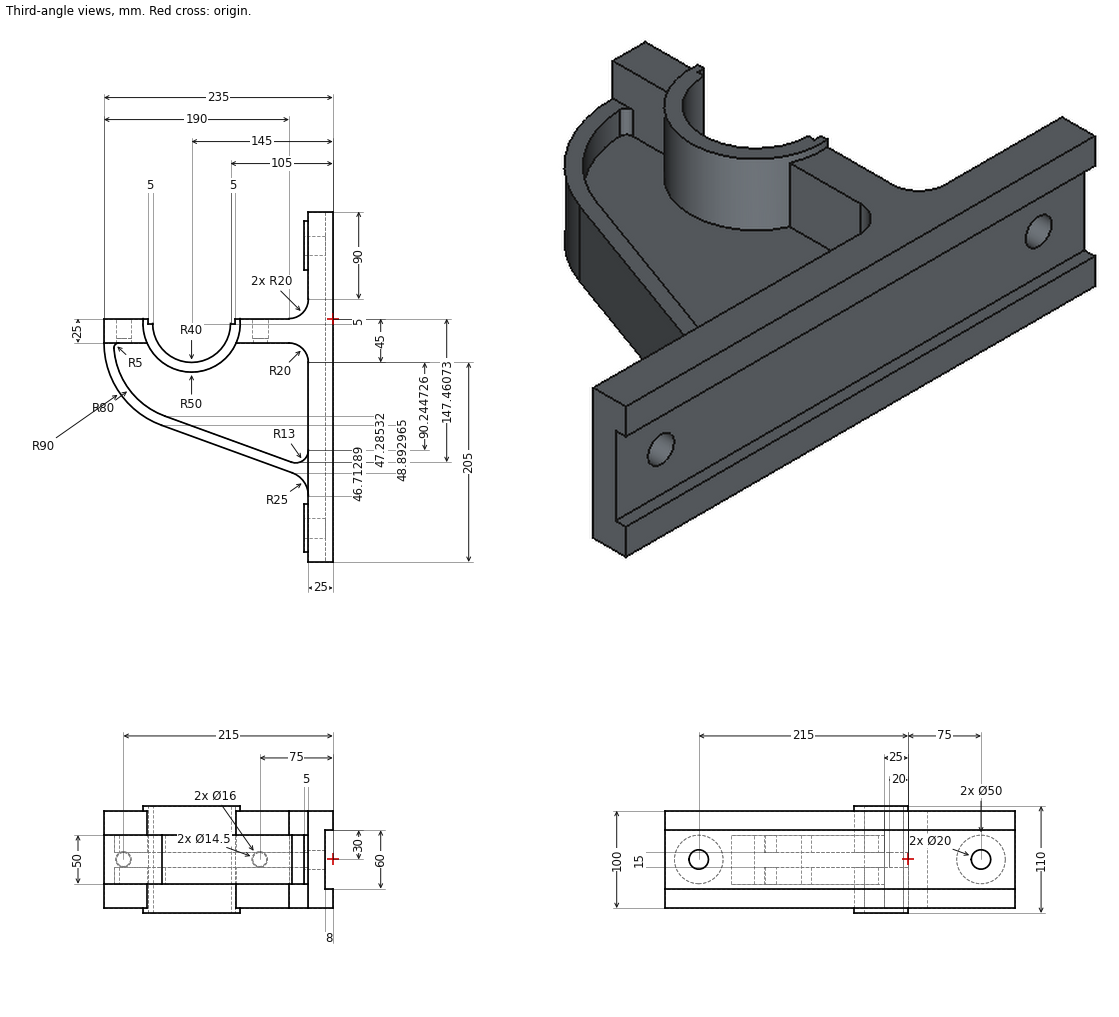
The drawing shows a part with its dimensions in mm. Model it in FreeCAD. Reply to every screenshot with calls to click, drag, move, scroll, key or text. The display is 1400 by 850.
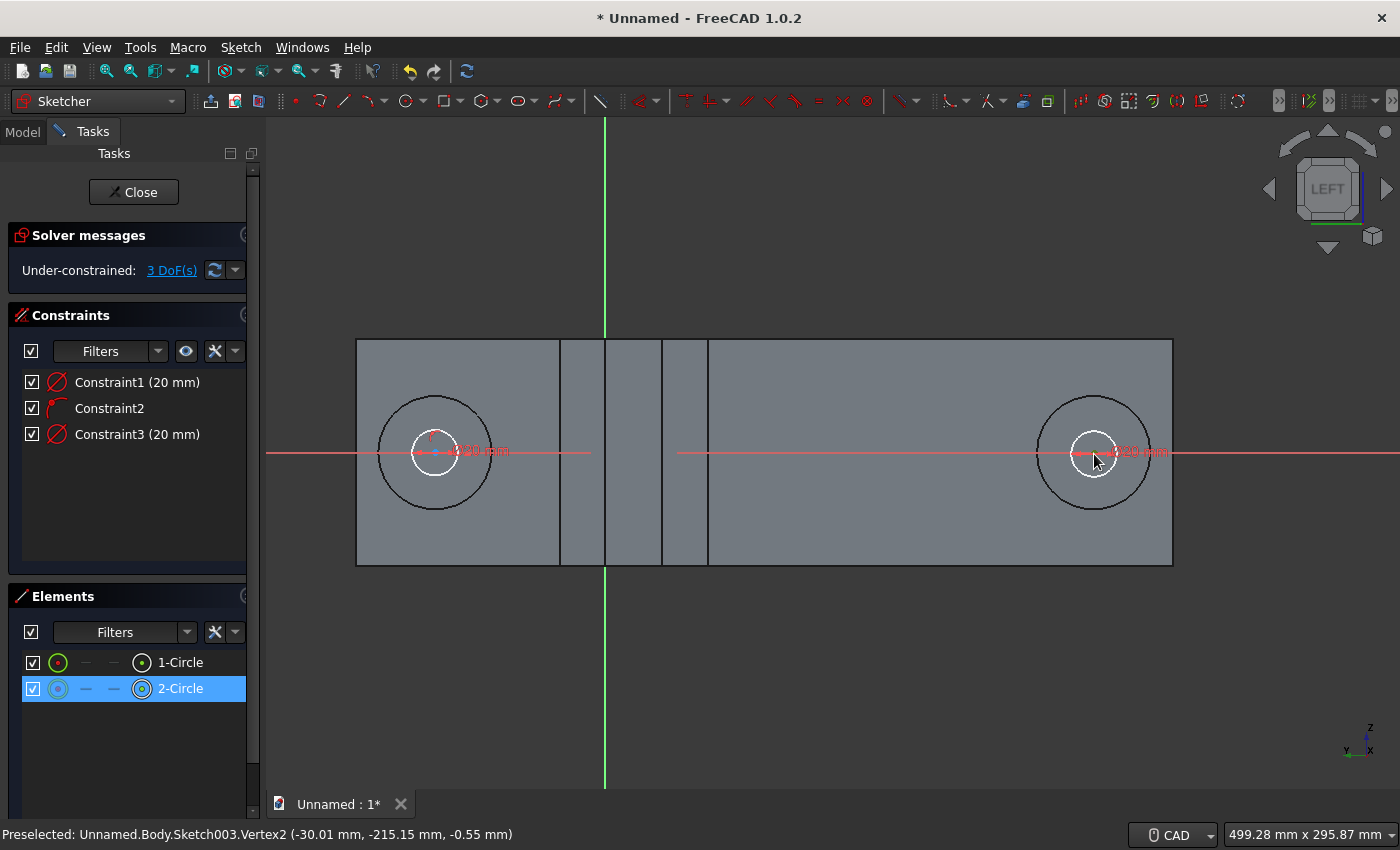
click(361, 453)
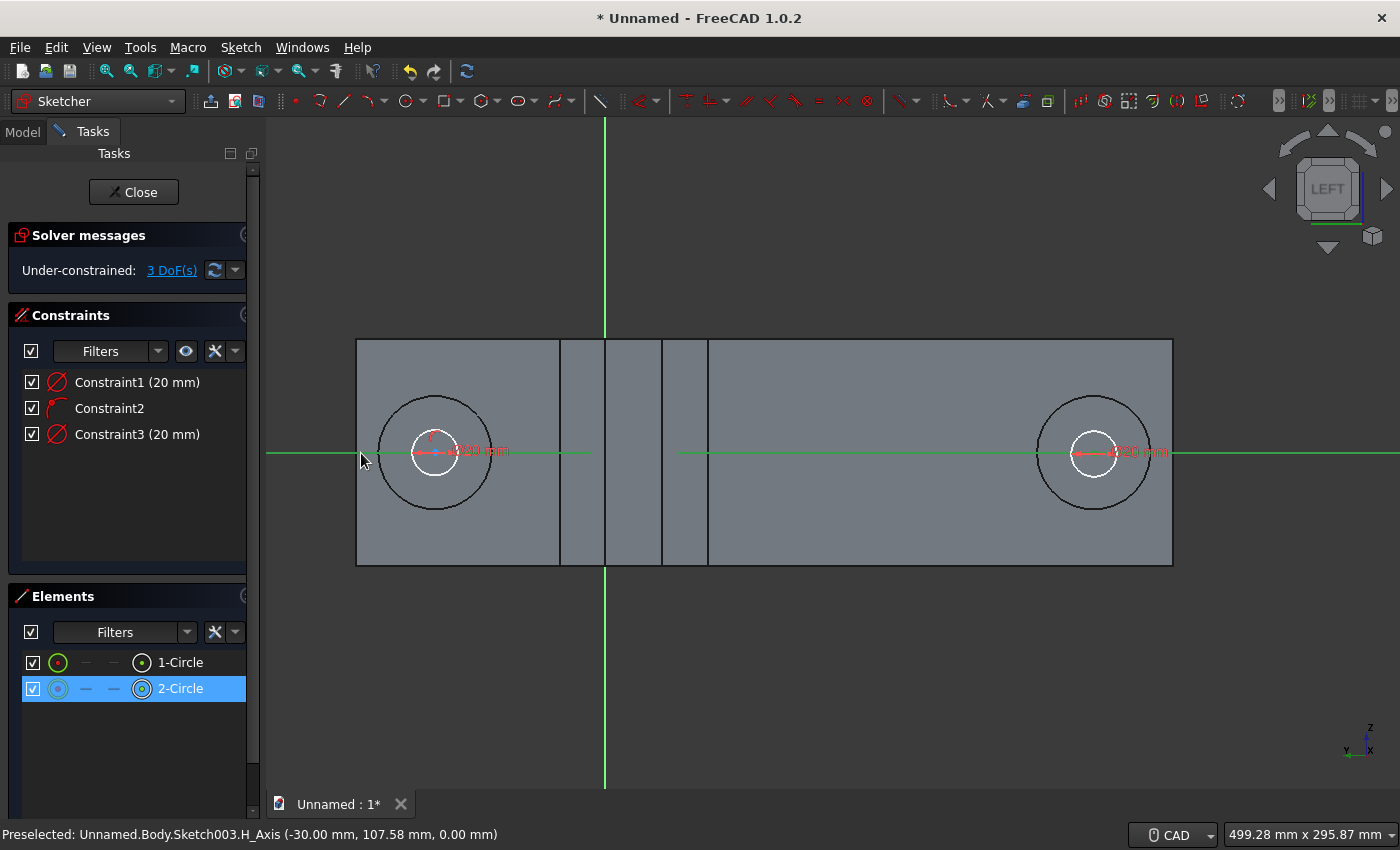
click(686, 102)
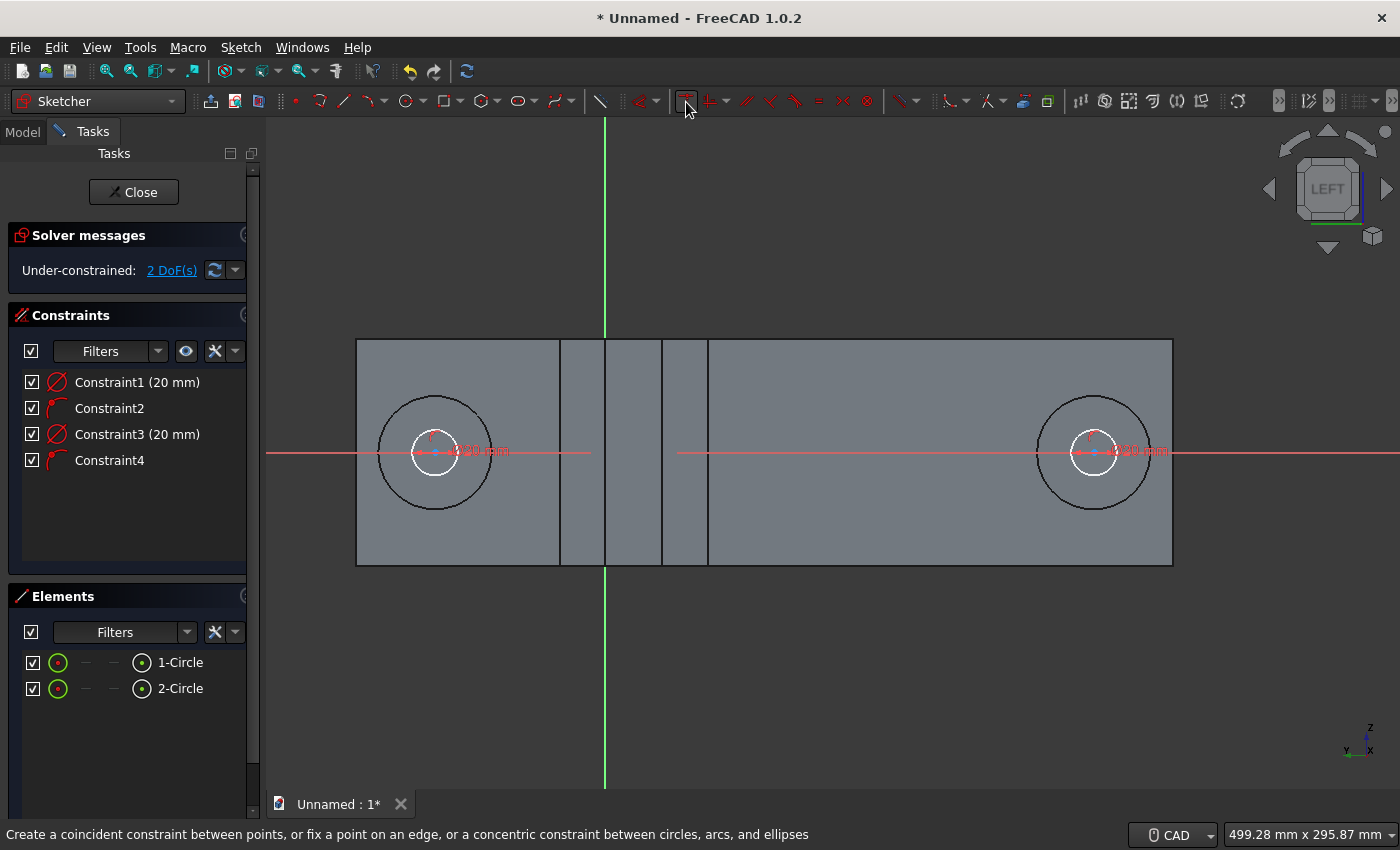
click(640, 102)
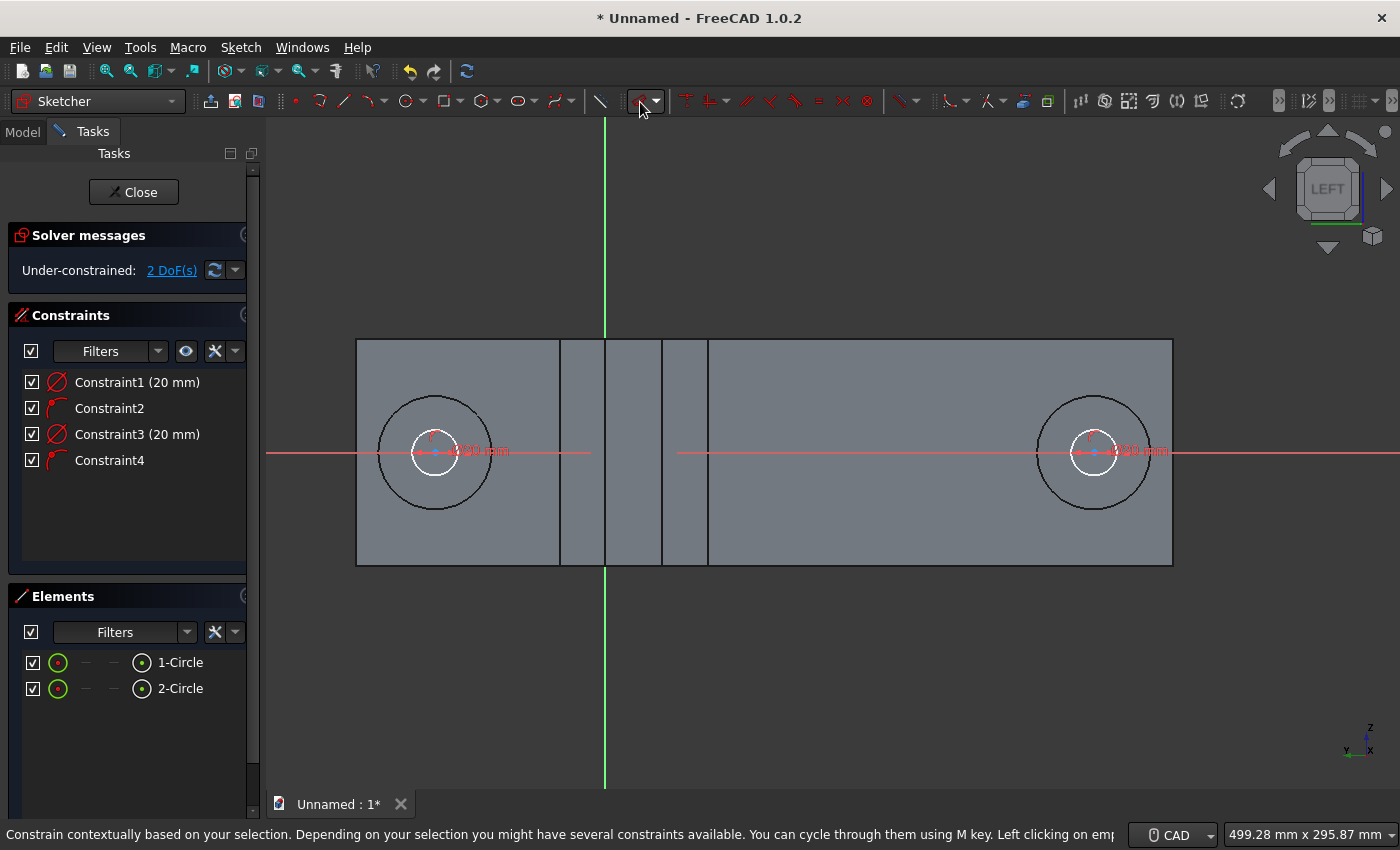
click(435, 453)
click(520, 487)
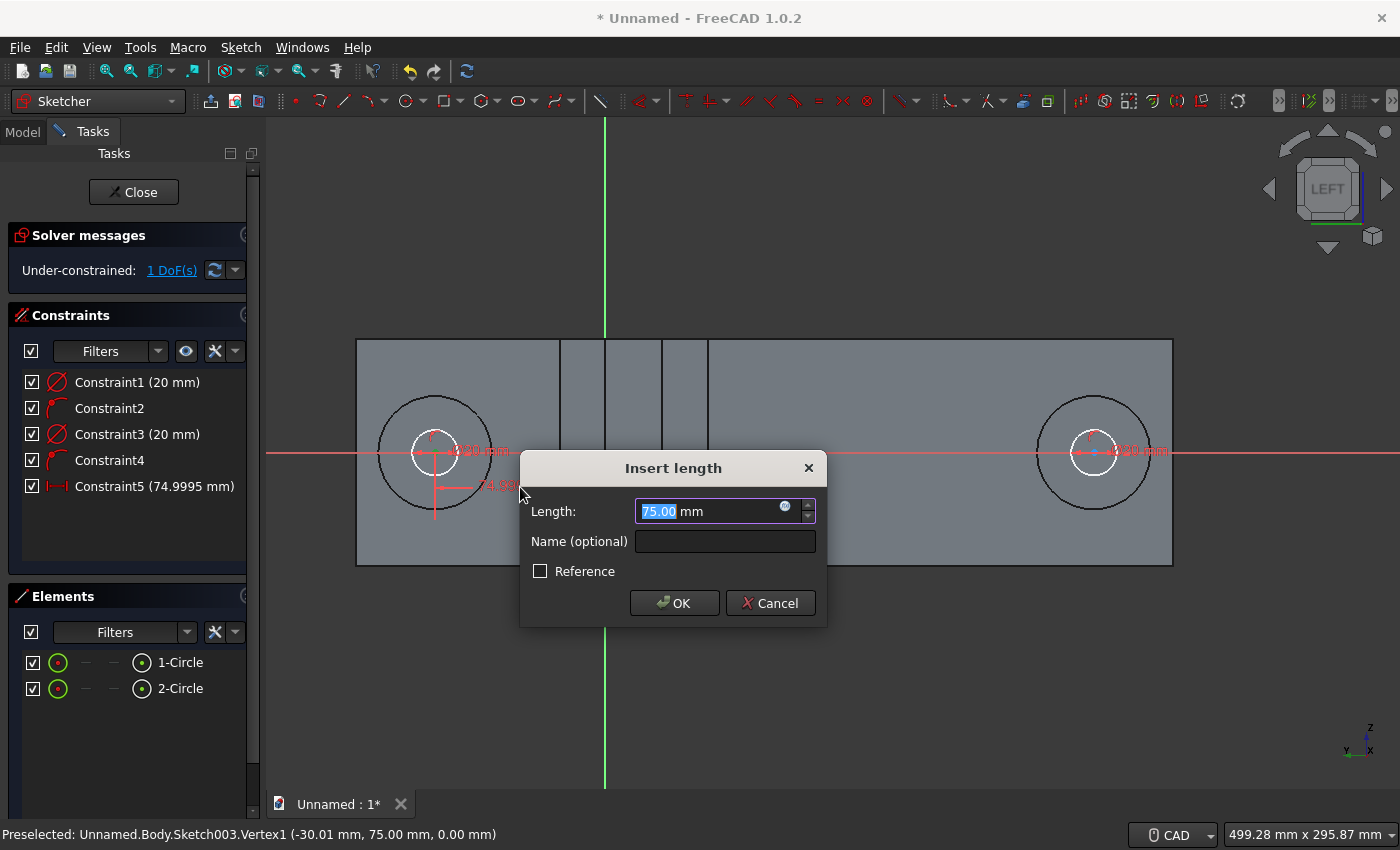
text(75)
key(Return)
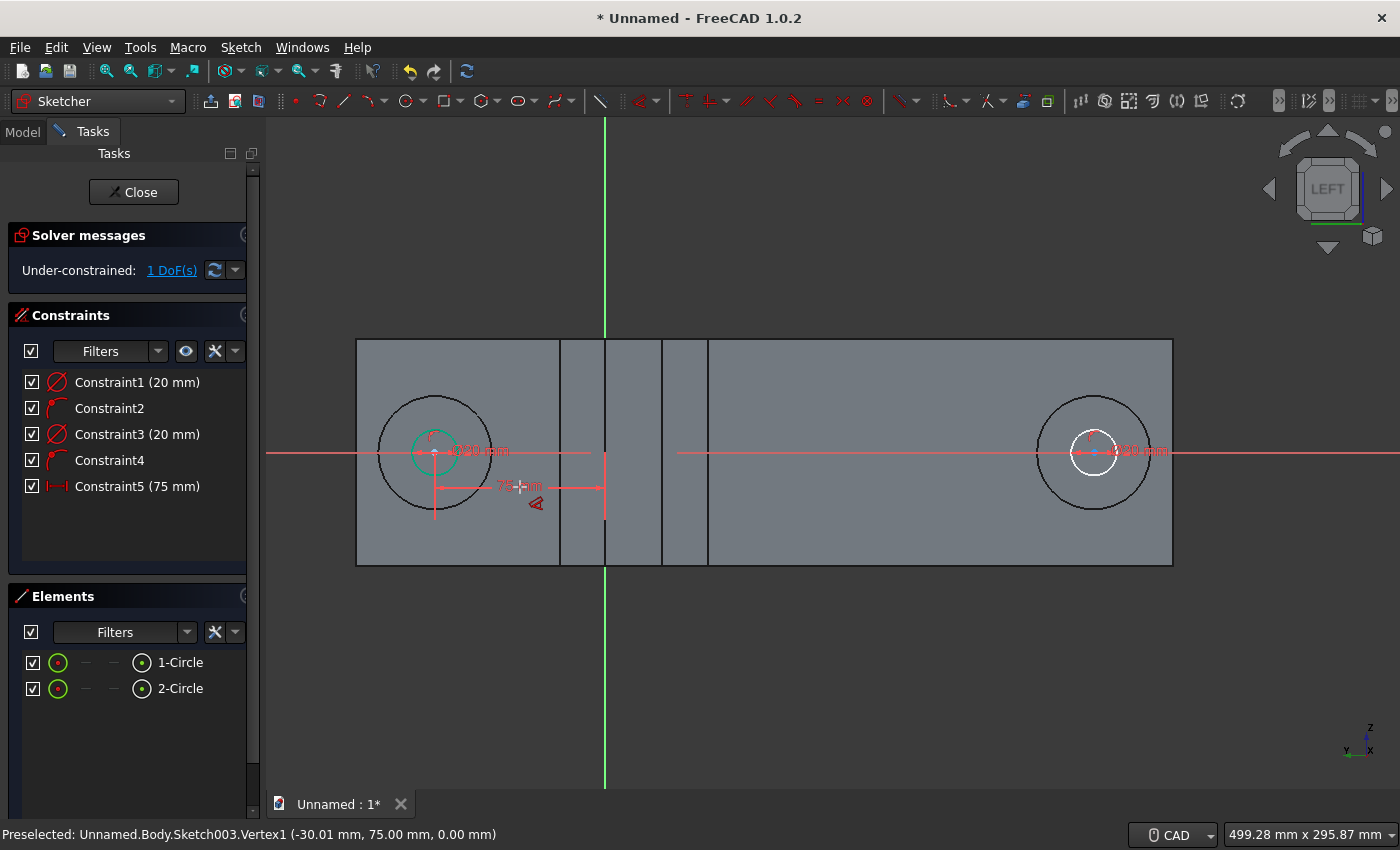
click(1094, 453)
click(850, 487)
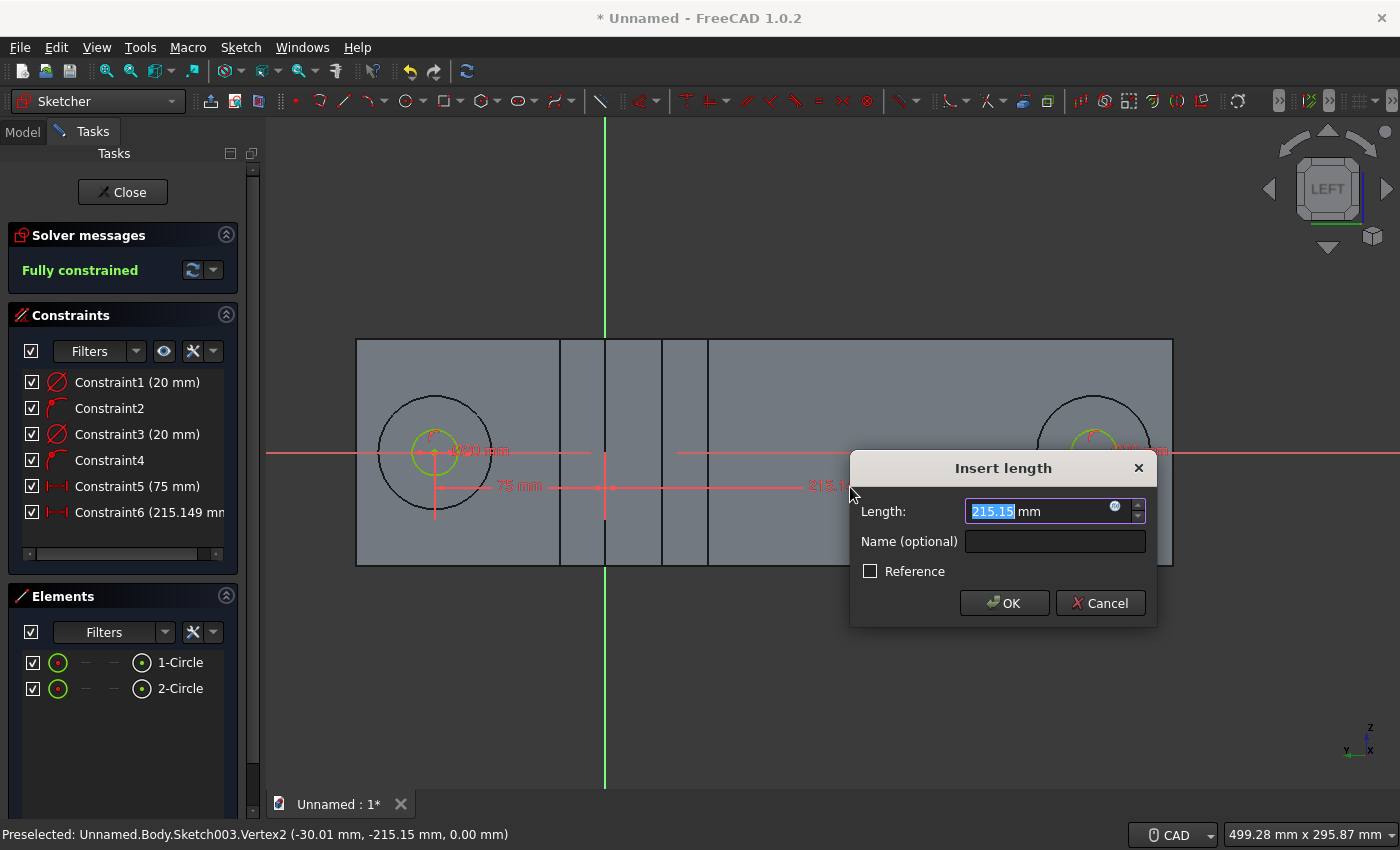
text(215)
key(Return)
key(Escape)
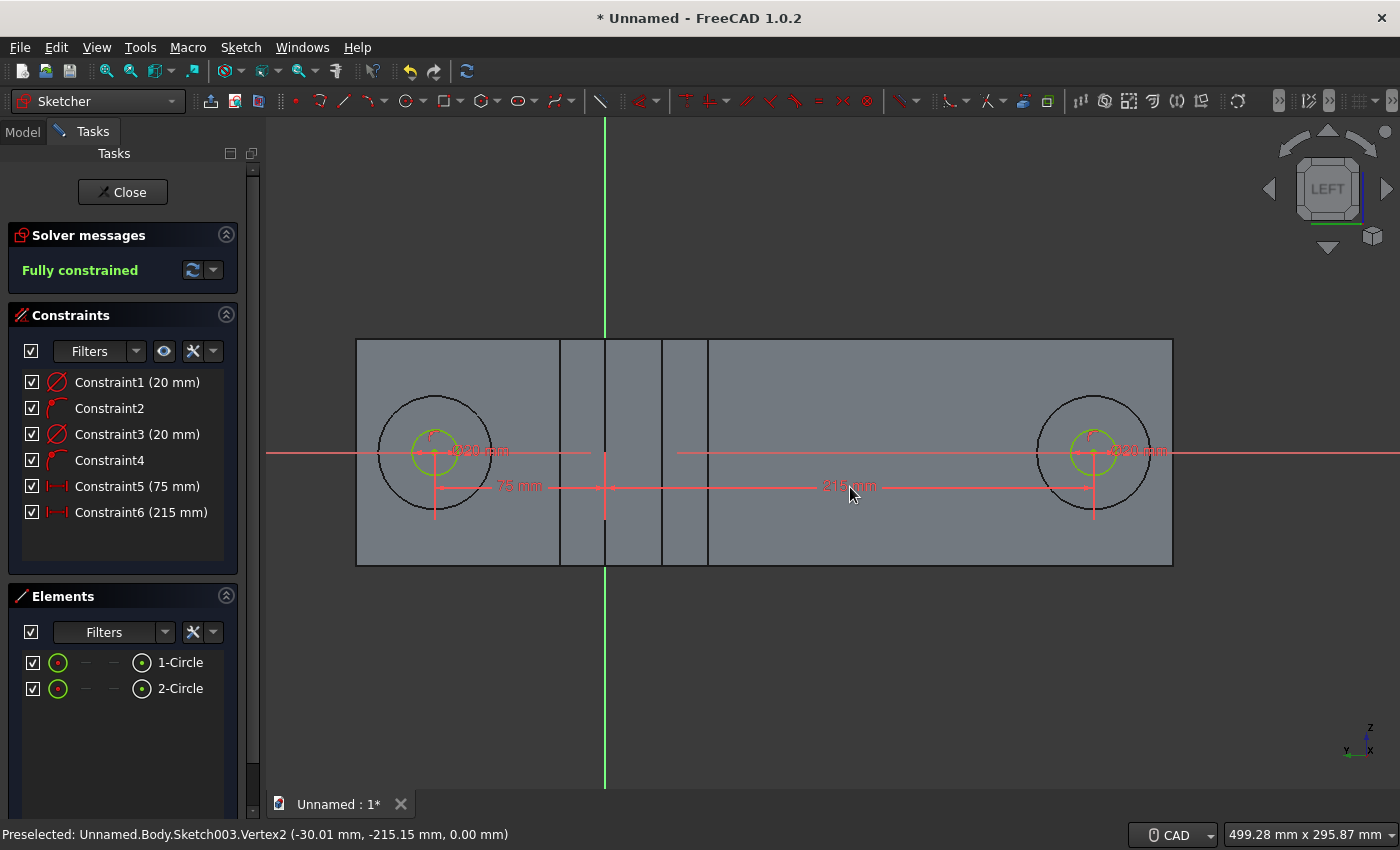
click(123, 192)